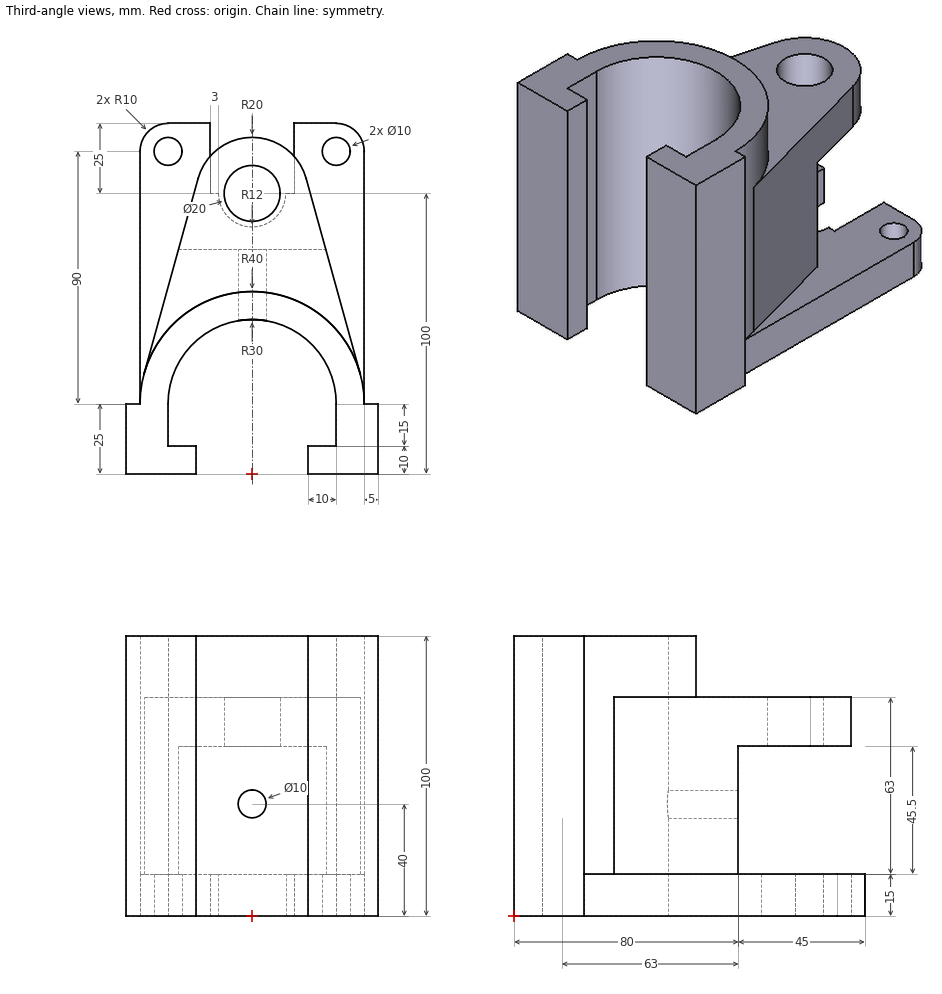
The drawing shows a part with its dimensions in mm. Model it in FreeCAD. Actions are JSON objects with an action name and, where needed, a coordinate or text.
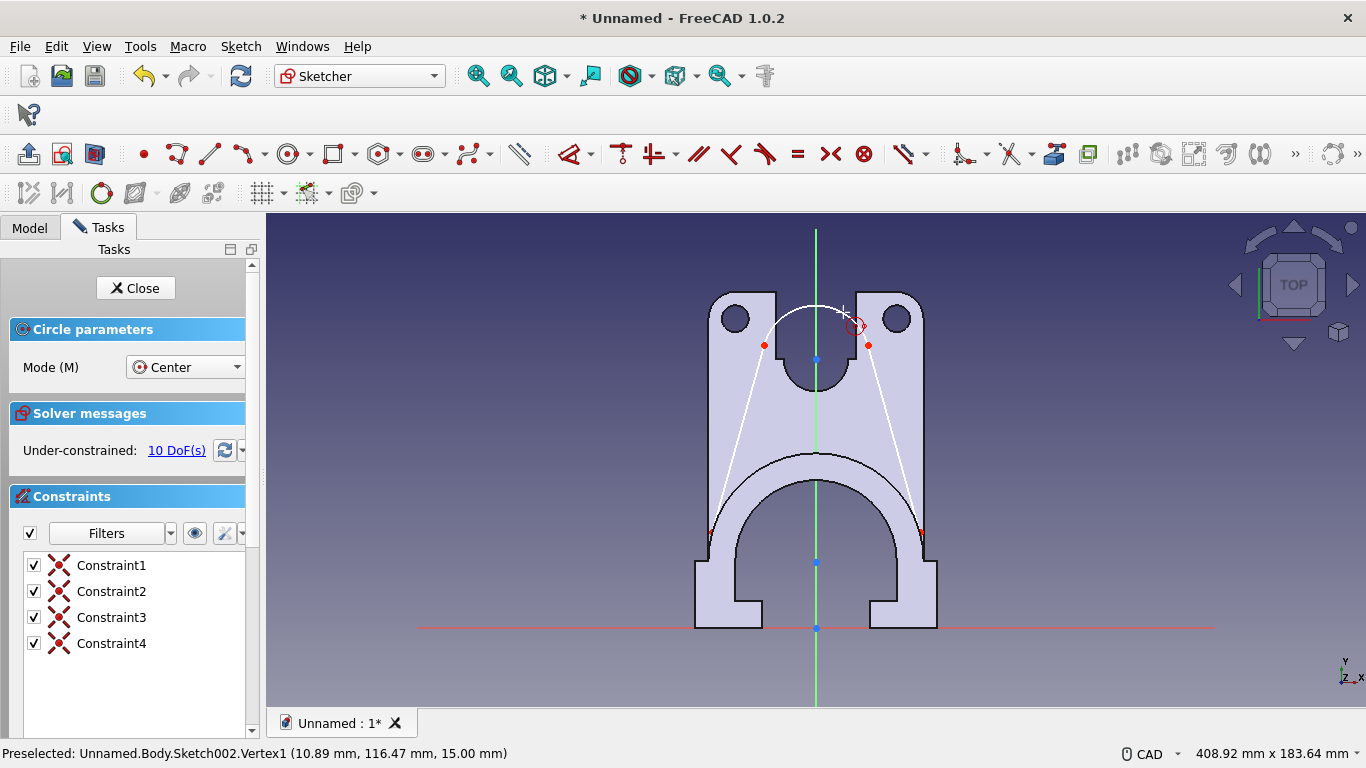
{"action": "left_click", "coordinate": [816, 359]}
{"action": "mouse_move", "coordinate": [835, 340]}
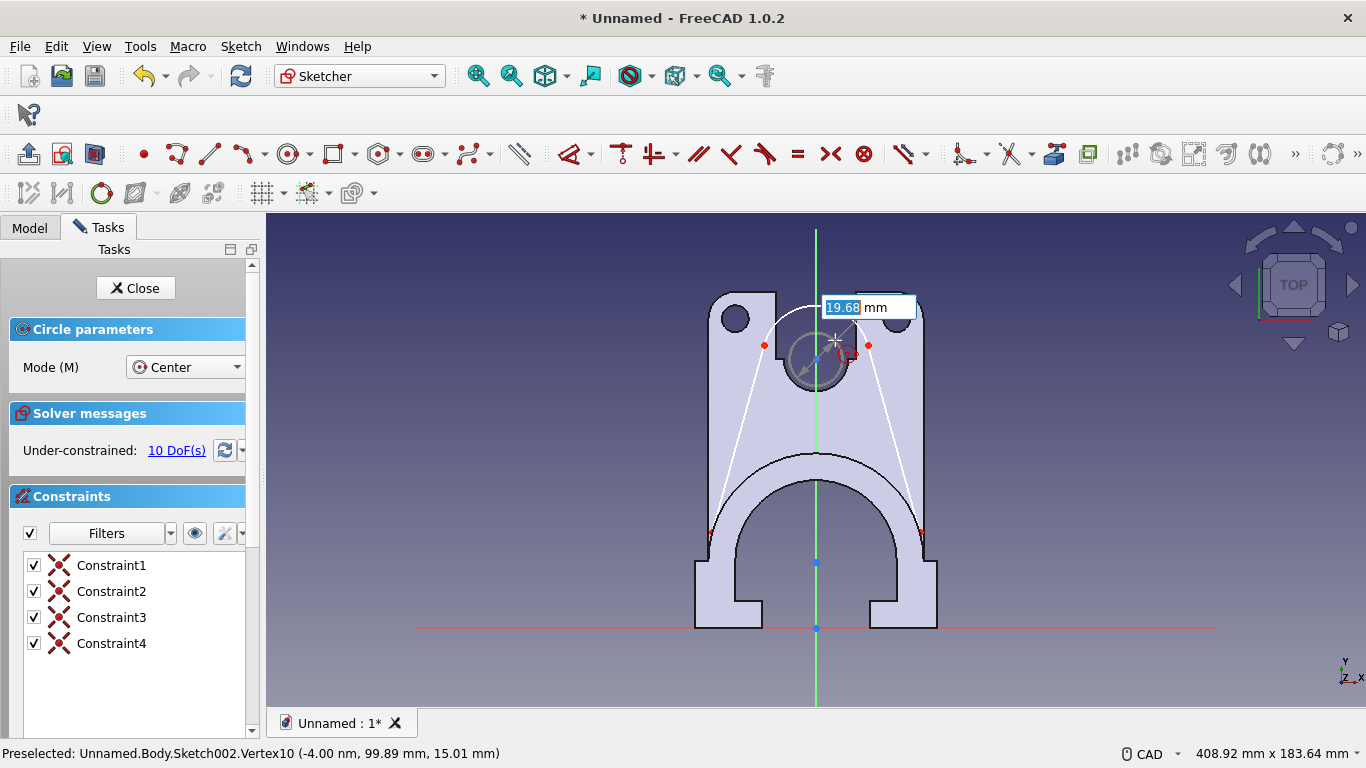
{"action": "type", "text": "20"}
{"action": "key", "text": "Return"}
{"action": "key", "text": "Escape"}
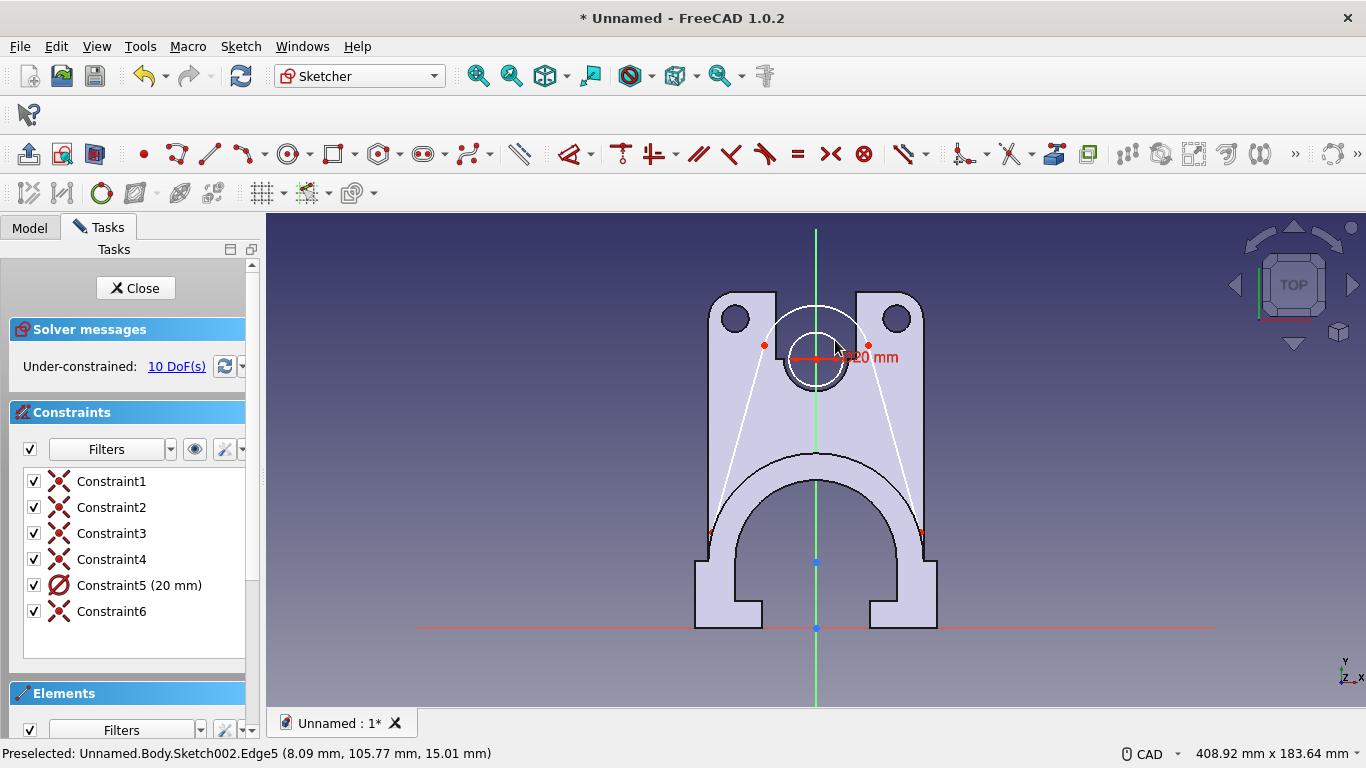
{"action": "left_click", "coordinate": [748, 402]}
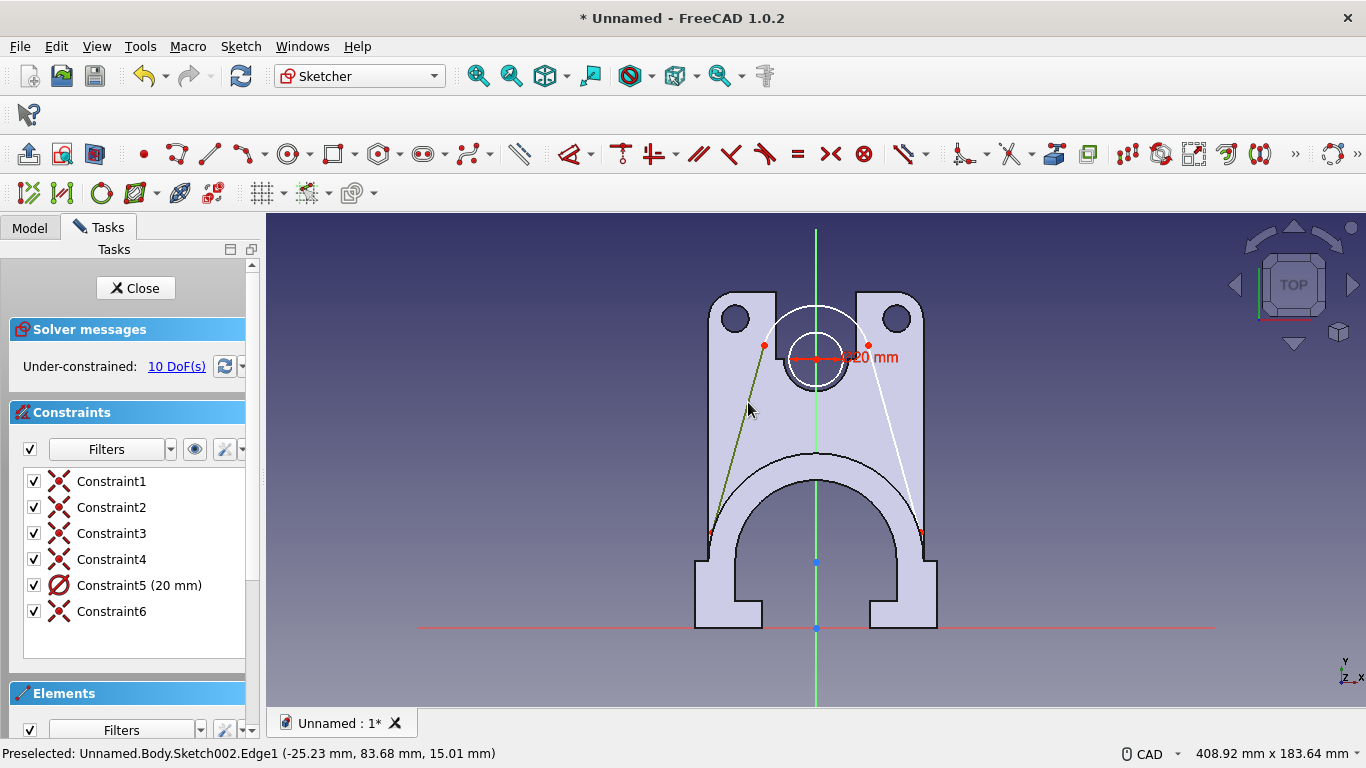
{"action": "left_click", "coordinate": [870, 468]}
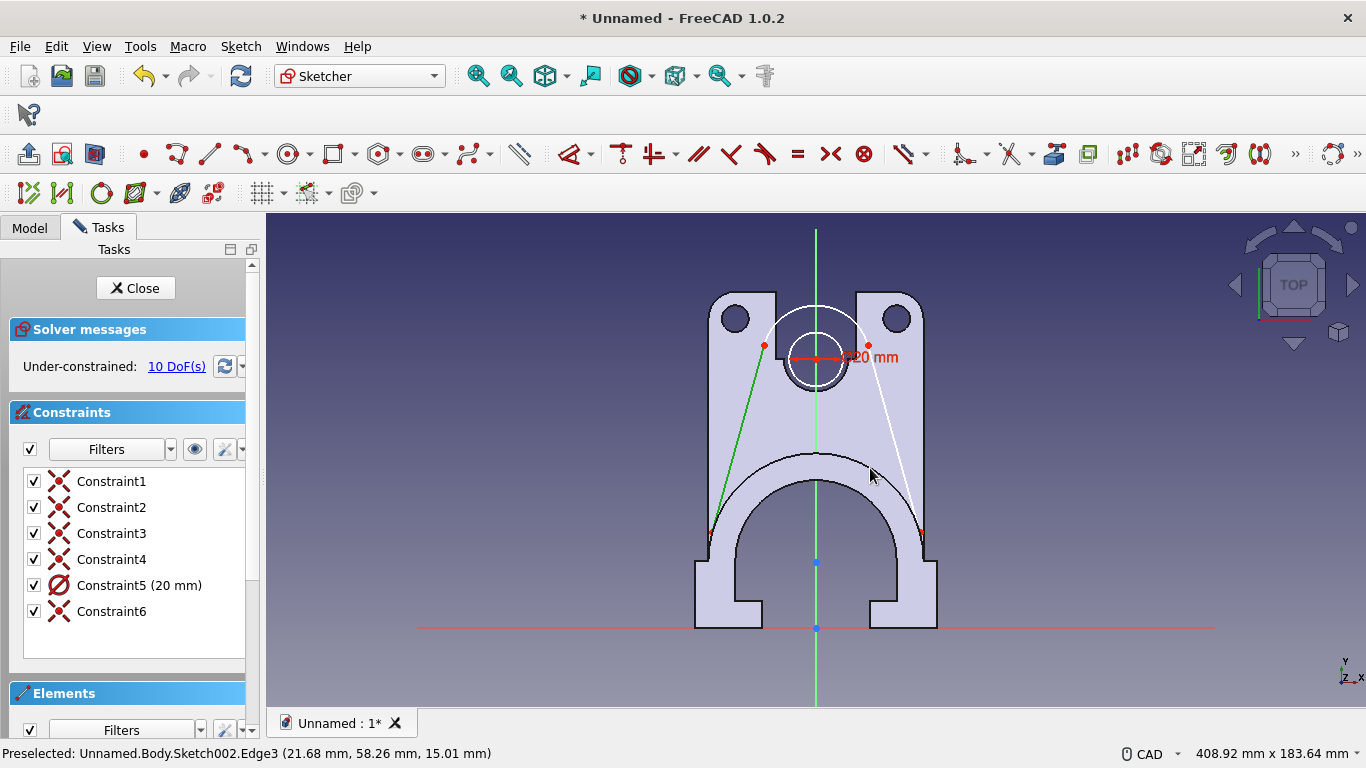
{"action": "key", "text": "t"}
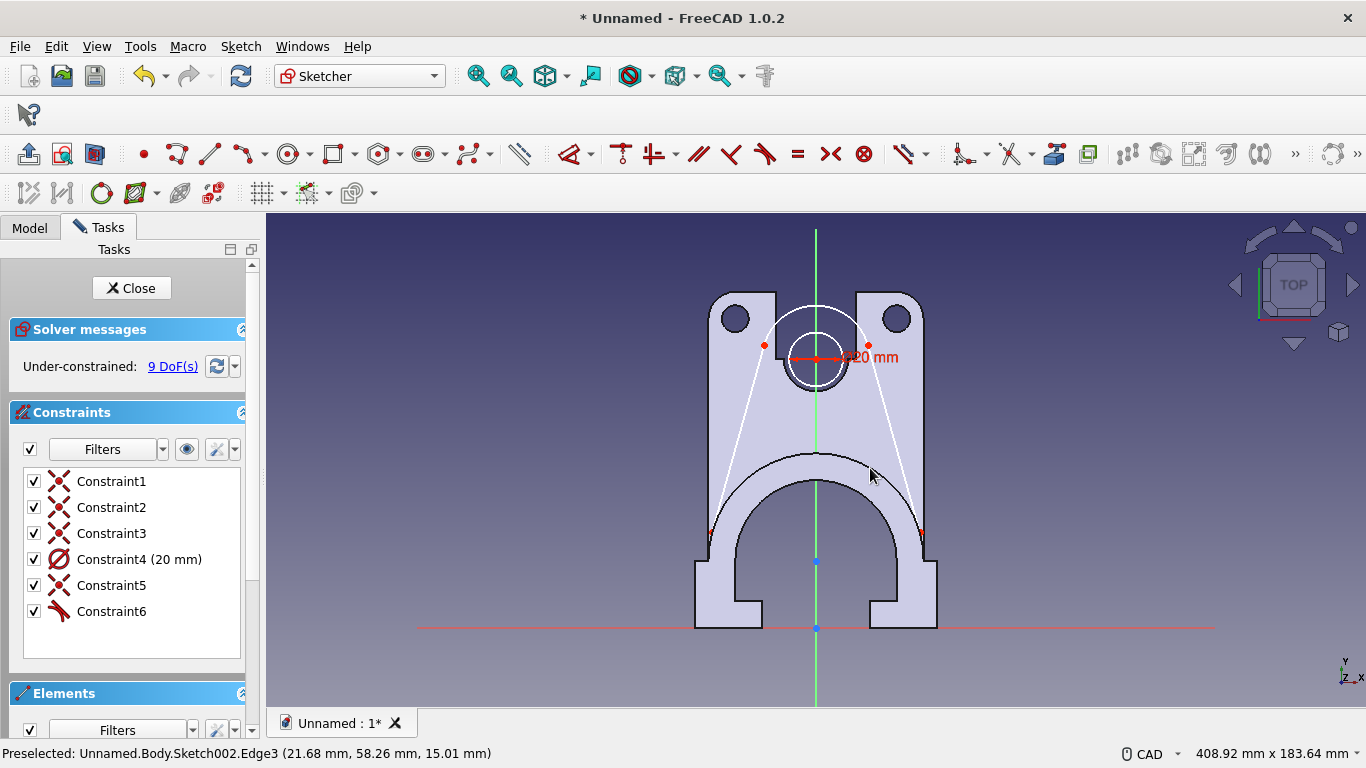
{"action": "left_click", "coordinate": [748, 402]}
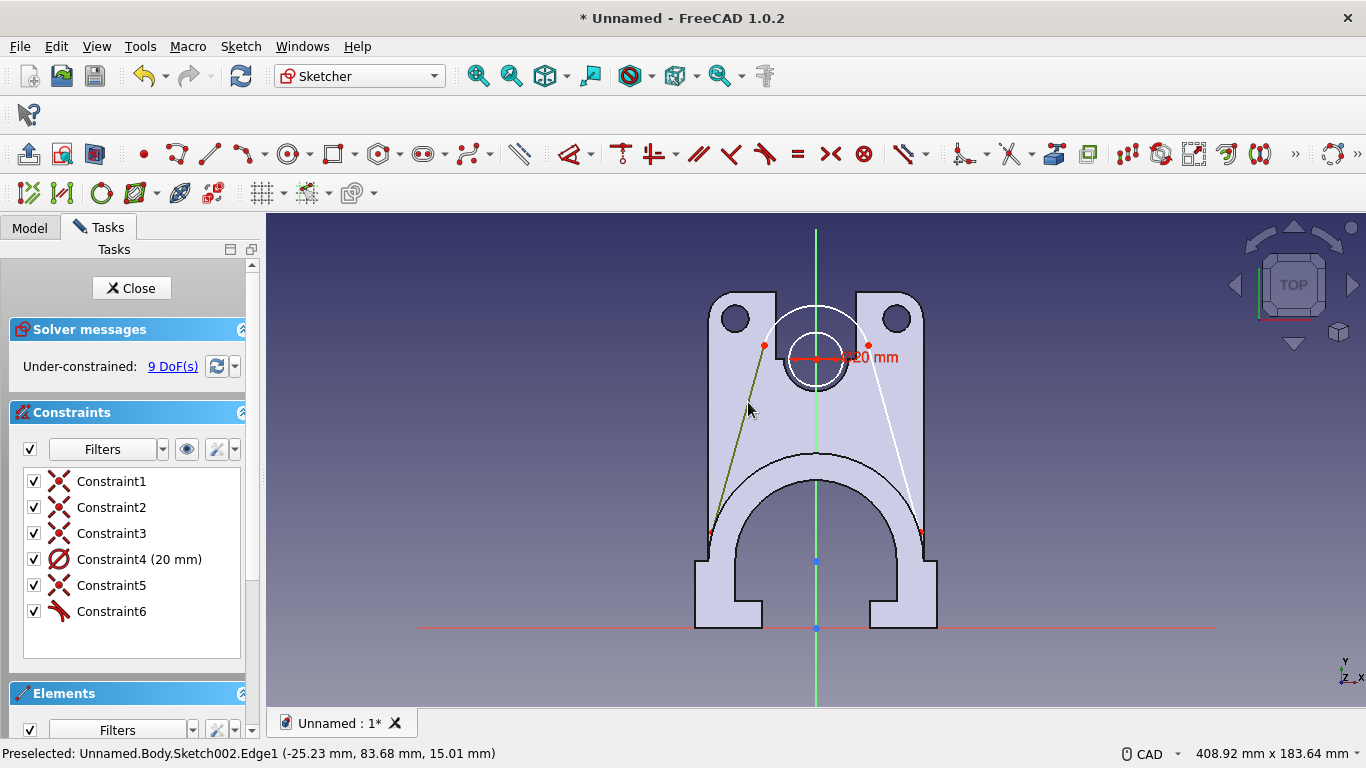
{"action": "left_click", "coordinate": [843, 313]}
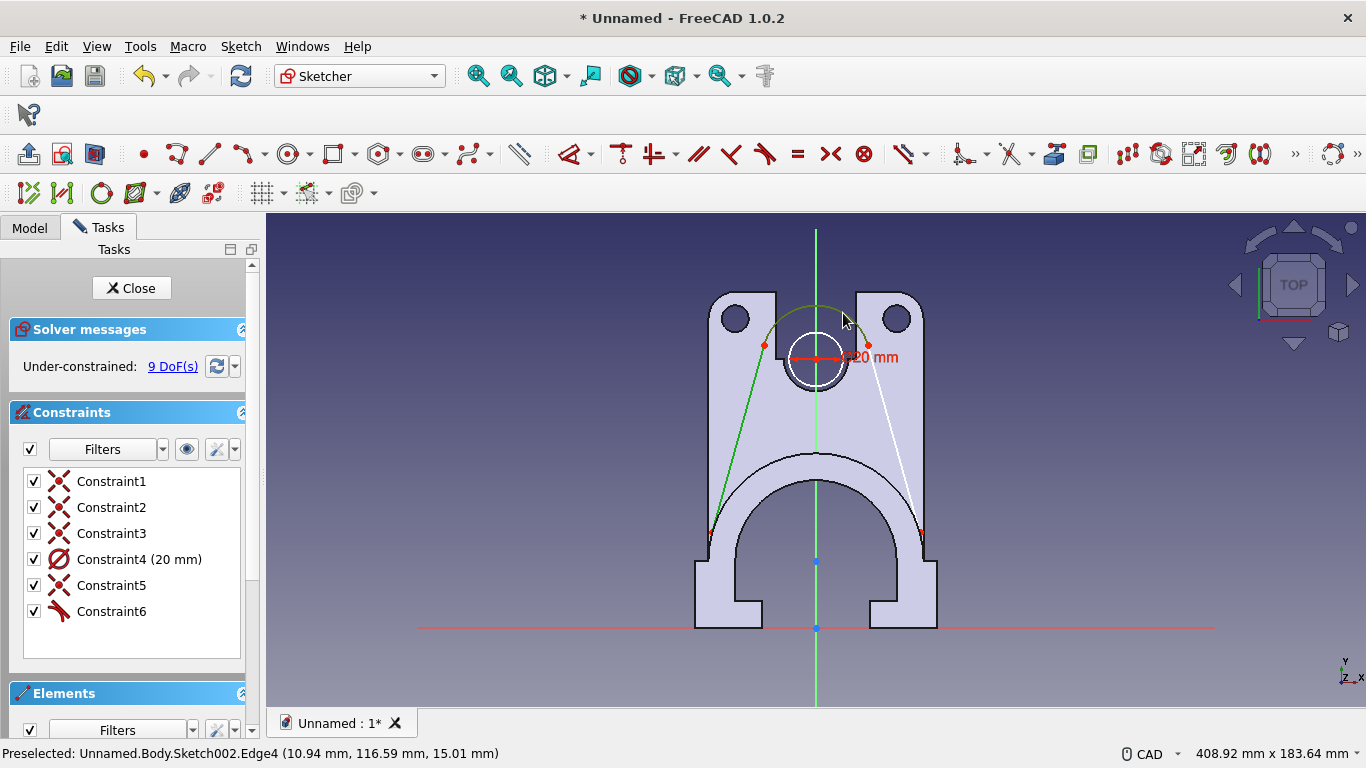
{"action": "key", "text": "t"}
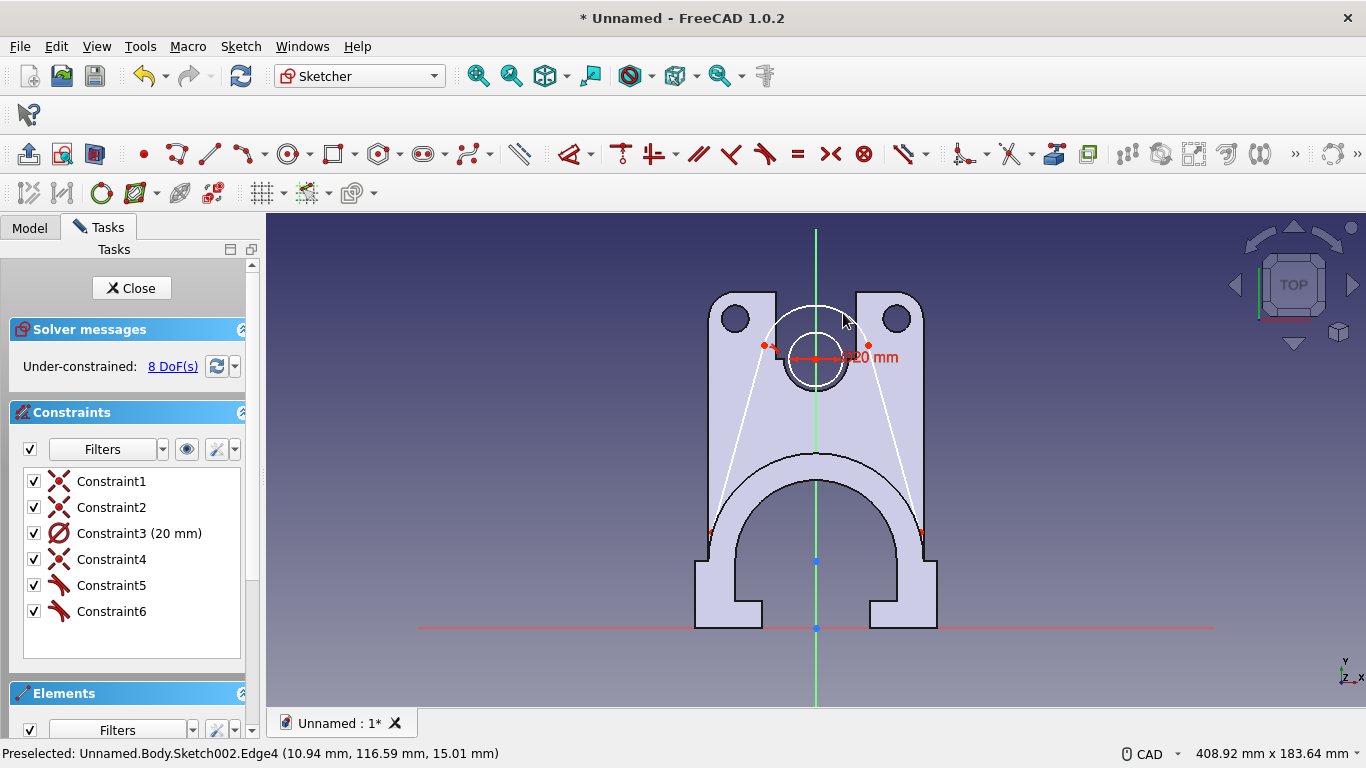
{"action": "left_click", "coordinate": [904, 477]}